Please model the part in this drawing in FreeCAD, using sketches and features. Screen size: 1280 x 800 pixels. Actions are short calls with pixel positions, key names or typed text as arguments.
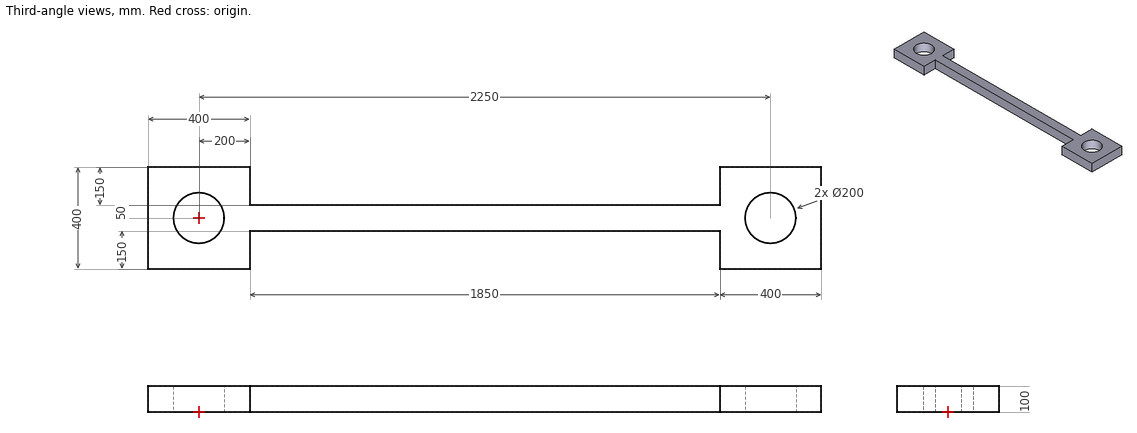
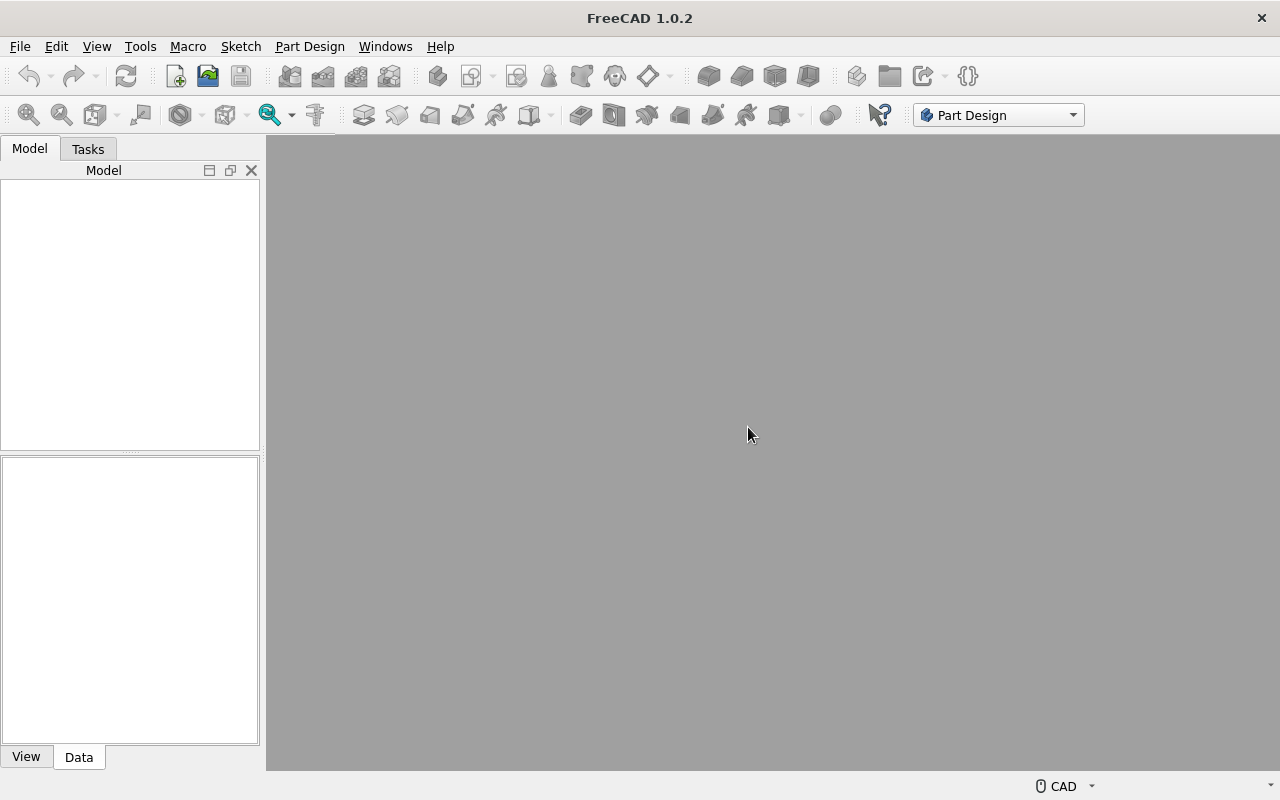
click(175, 76)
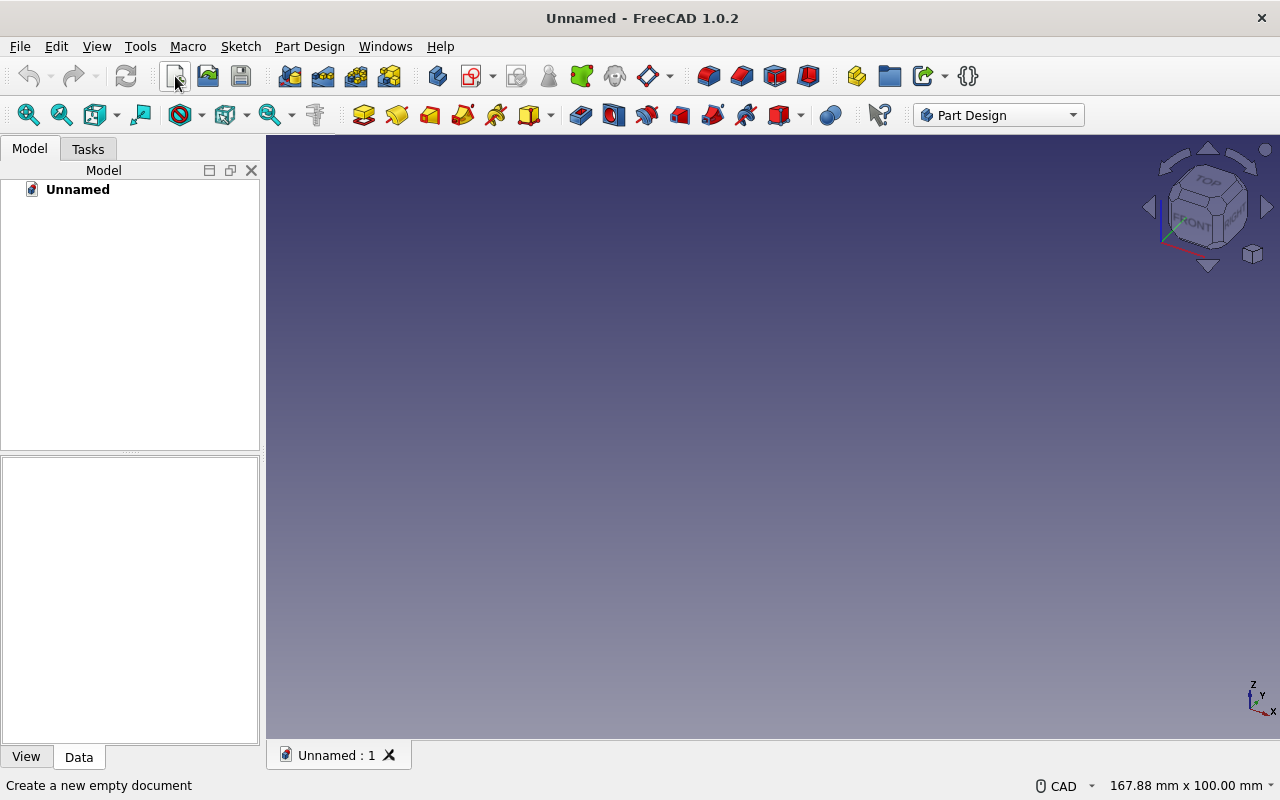
click(470, 76)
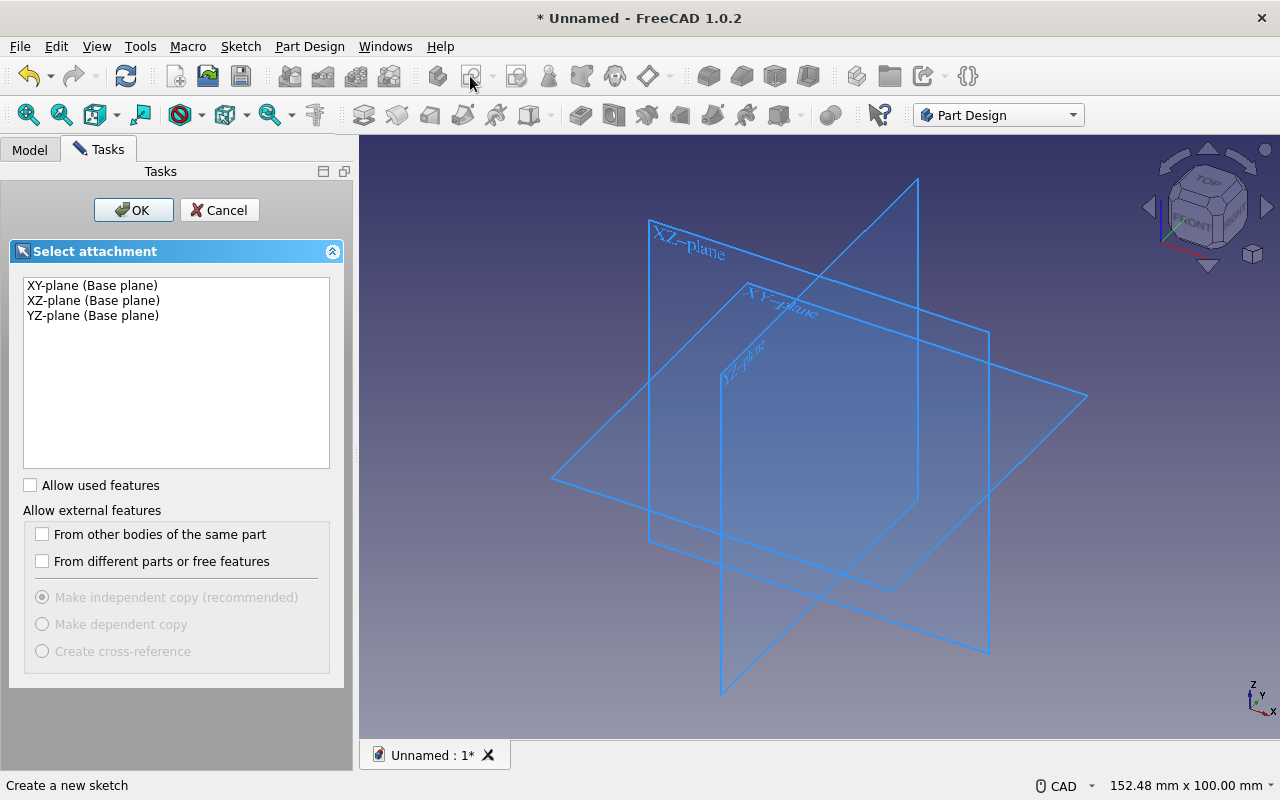
click(84, 286)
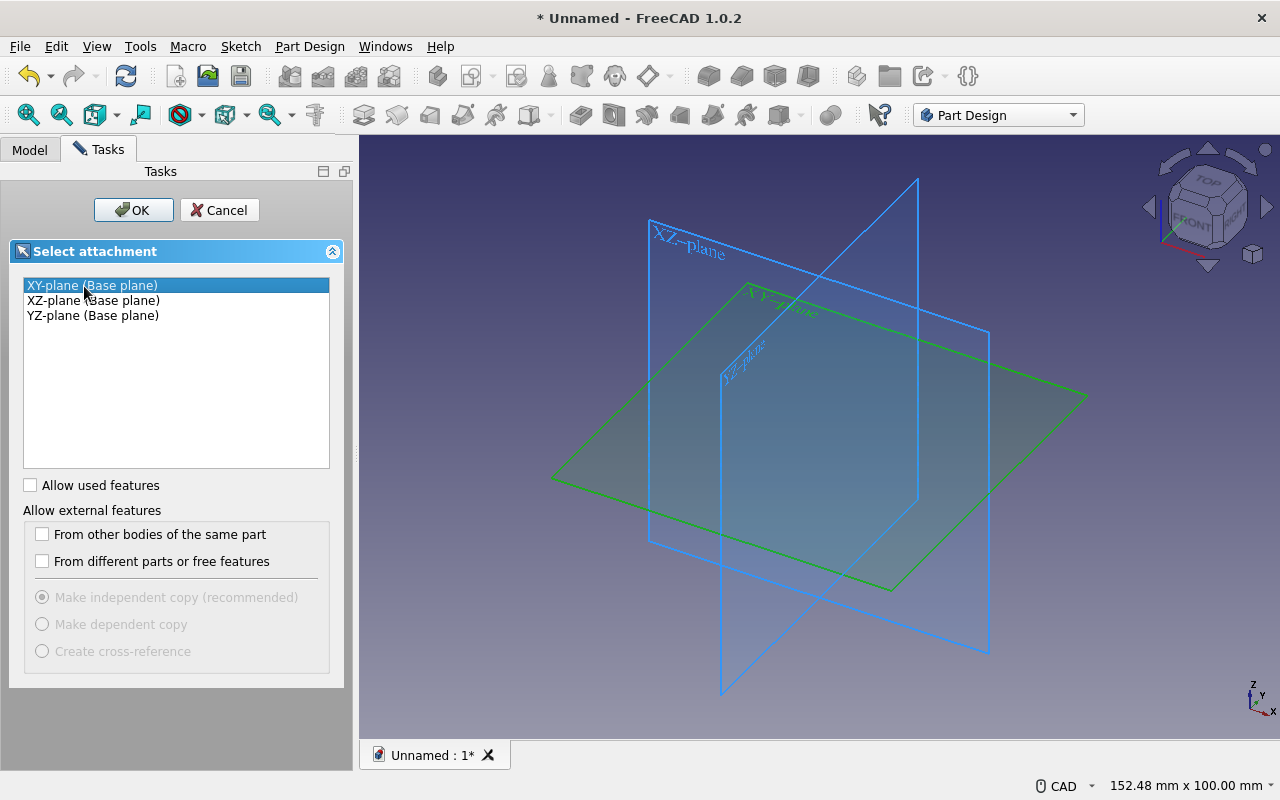
click(134, 210)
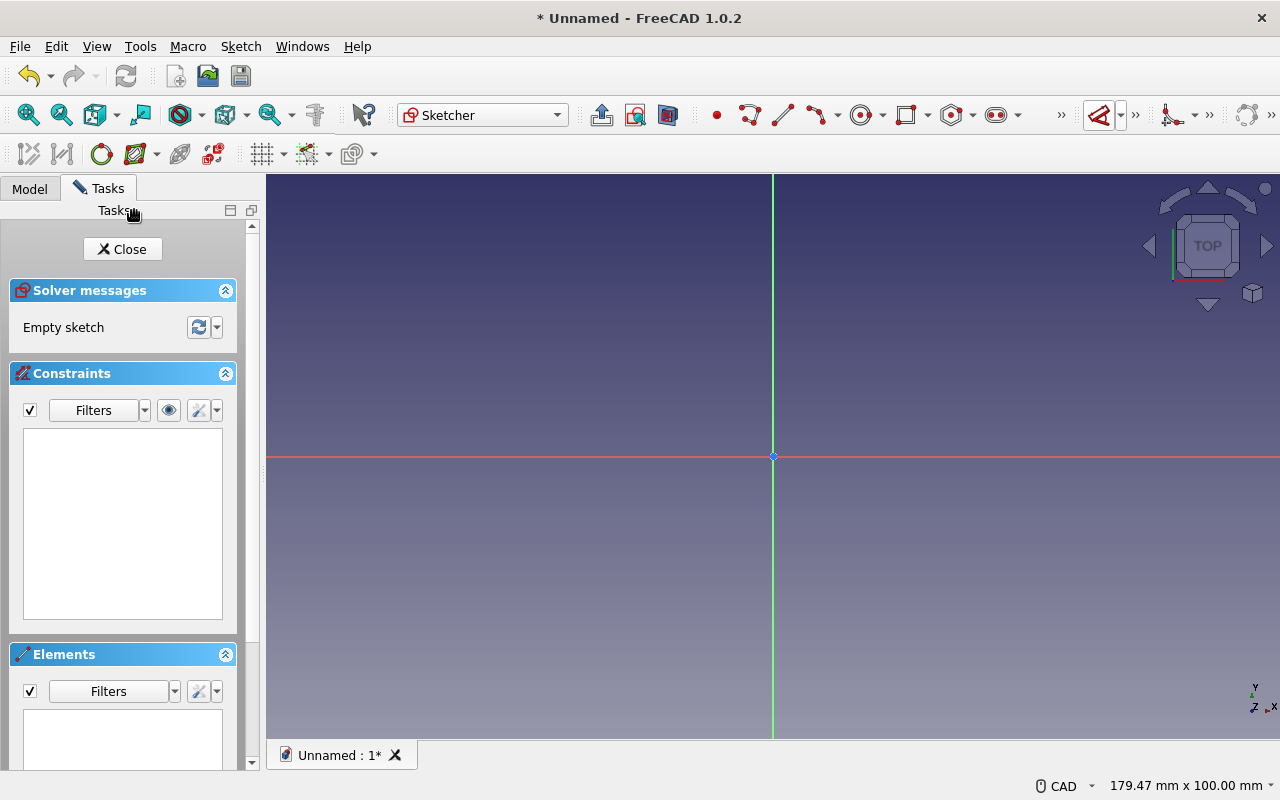
scroll(368, 457, down, 15)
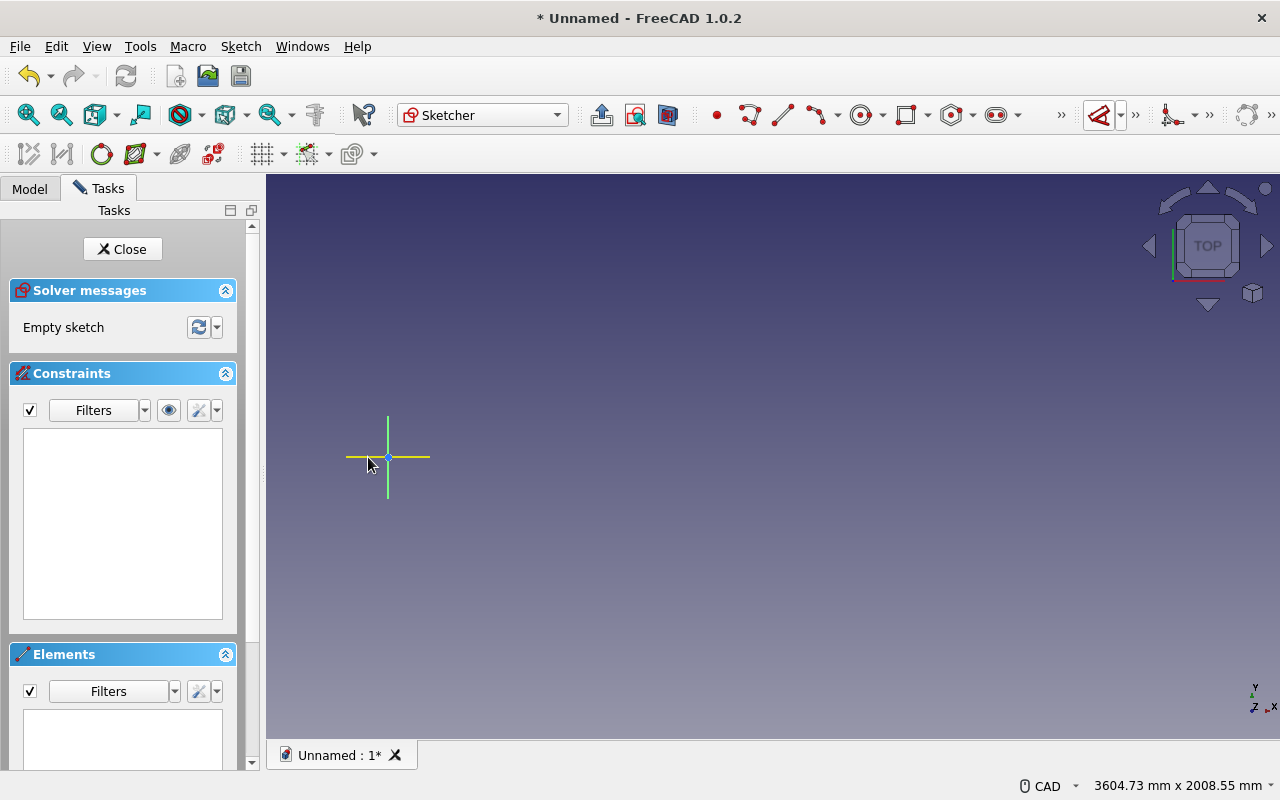
click(750, 116)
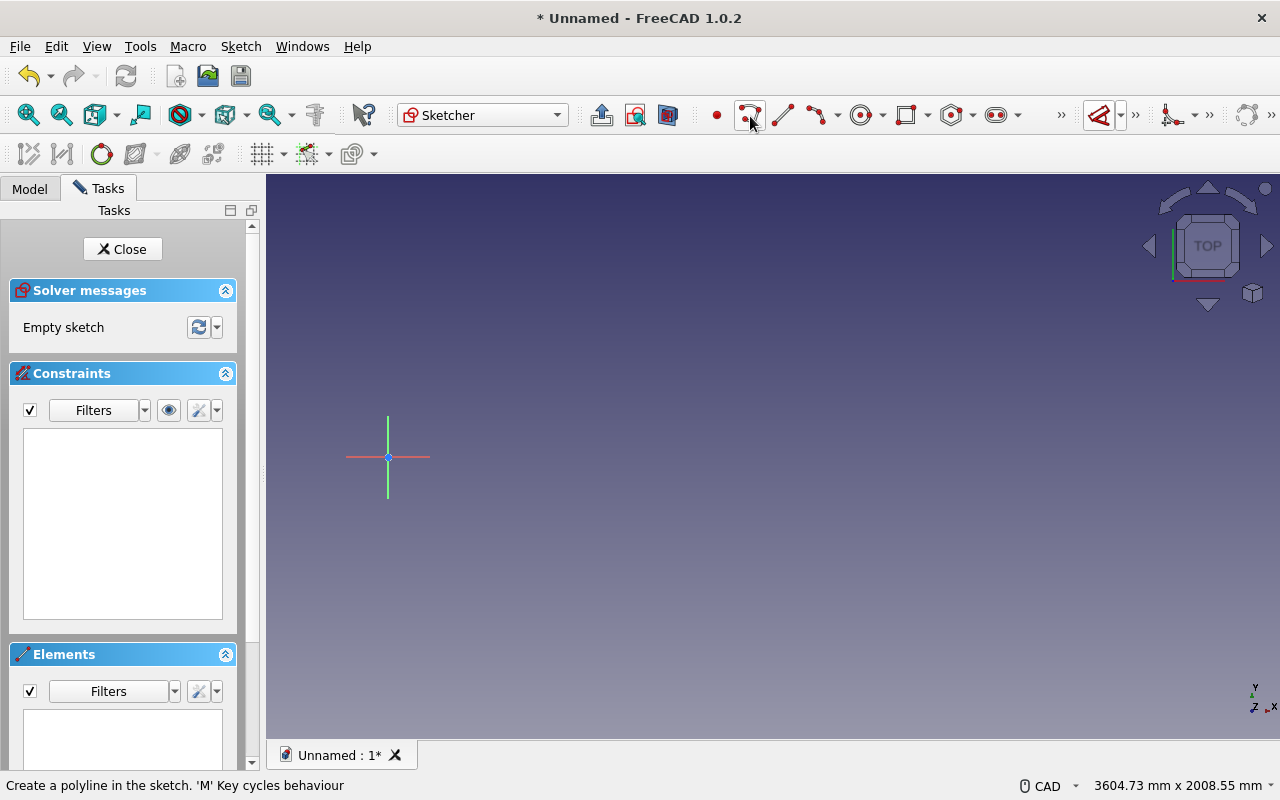
click(445, 443)
click(445, 401)
click(332, 401)
click(332, 514)
click(445, 514)
click(445, 472)
click(965, 472)
click(965, 514)
click(1077, 514)
click(1077, 401)
click(965, 401)
click(965, 443)
click(445, 444)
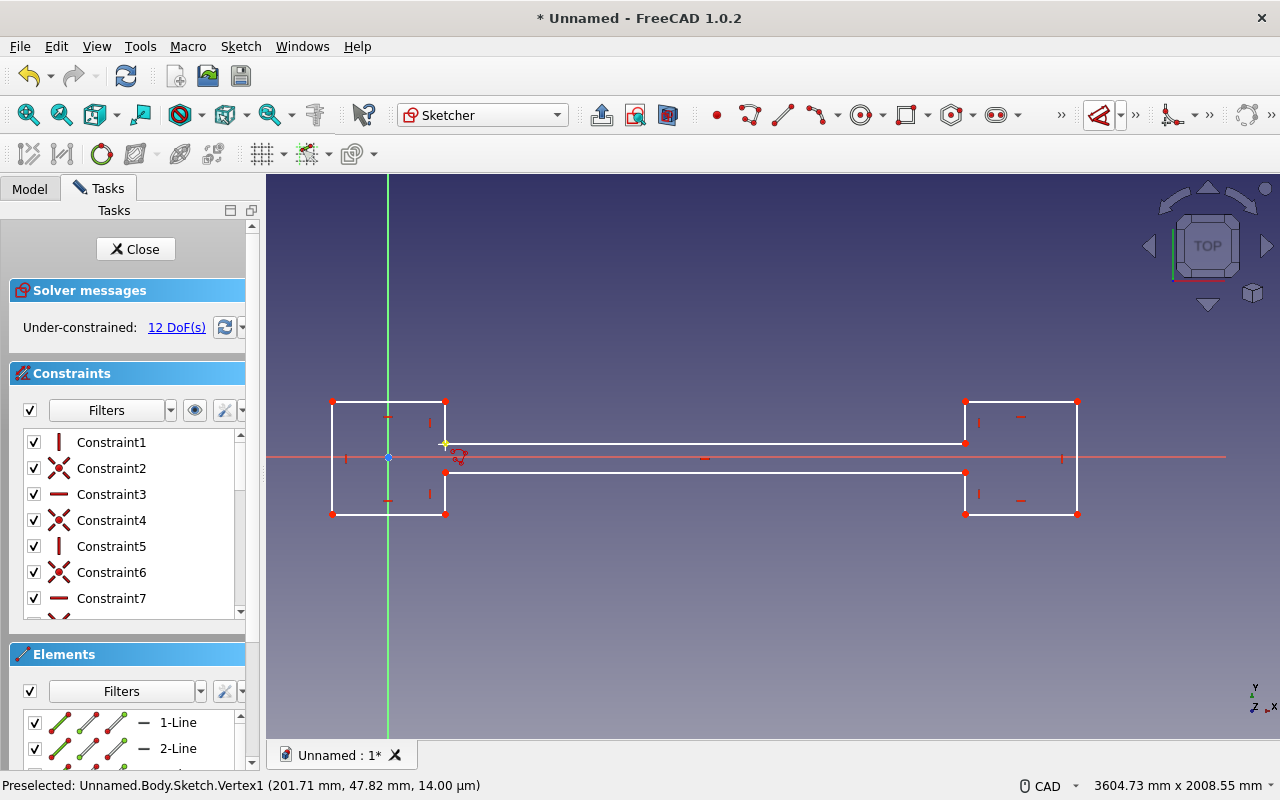
click(860, 116)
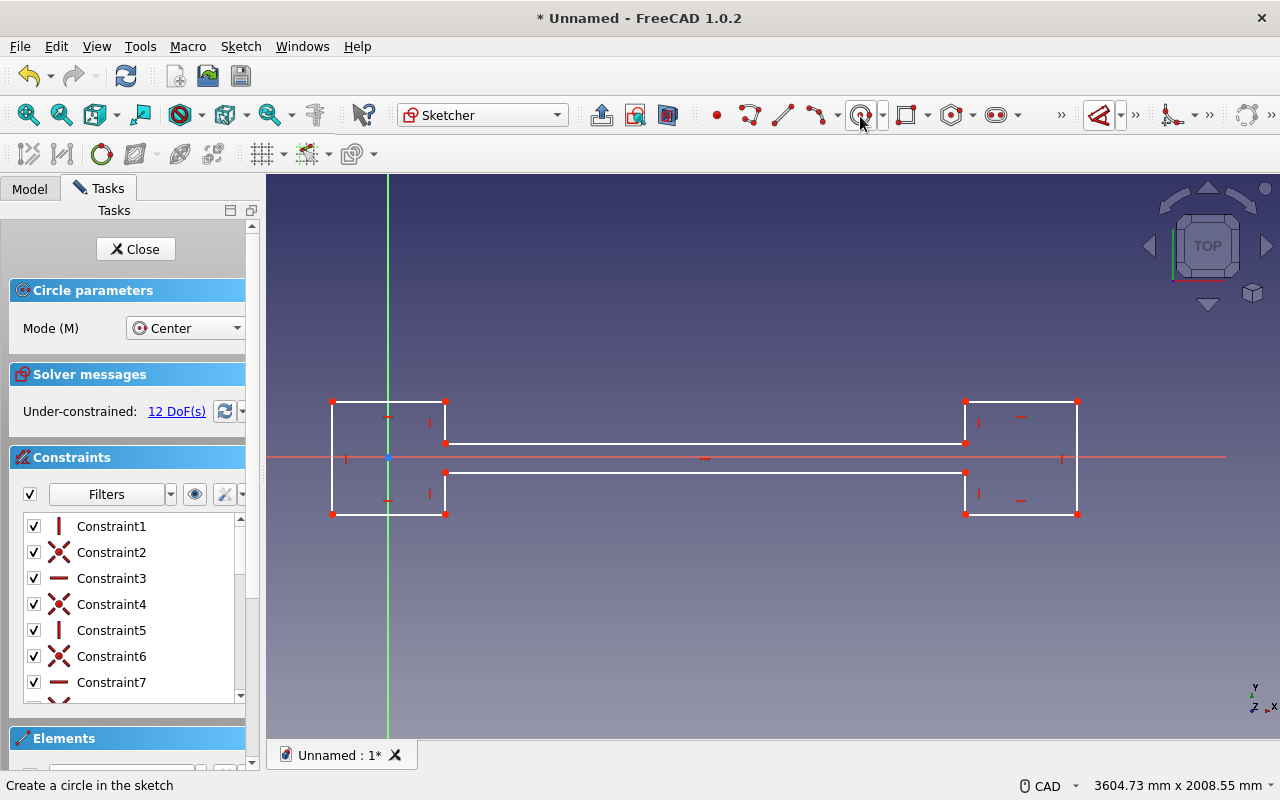
click(1021, 457)
click(1041, 438)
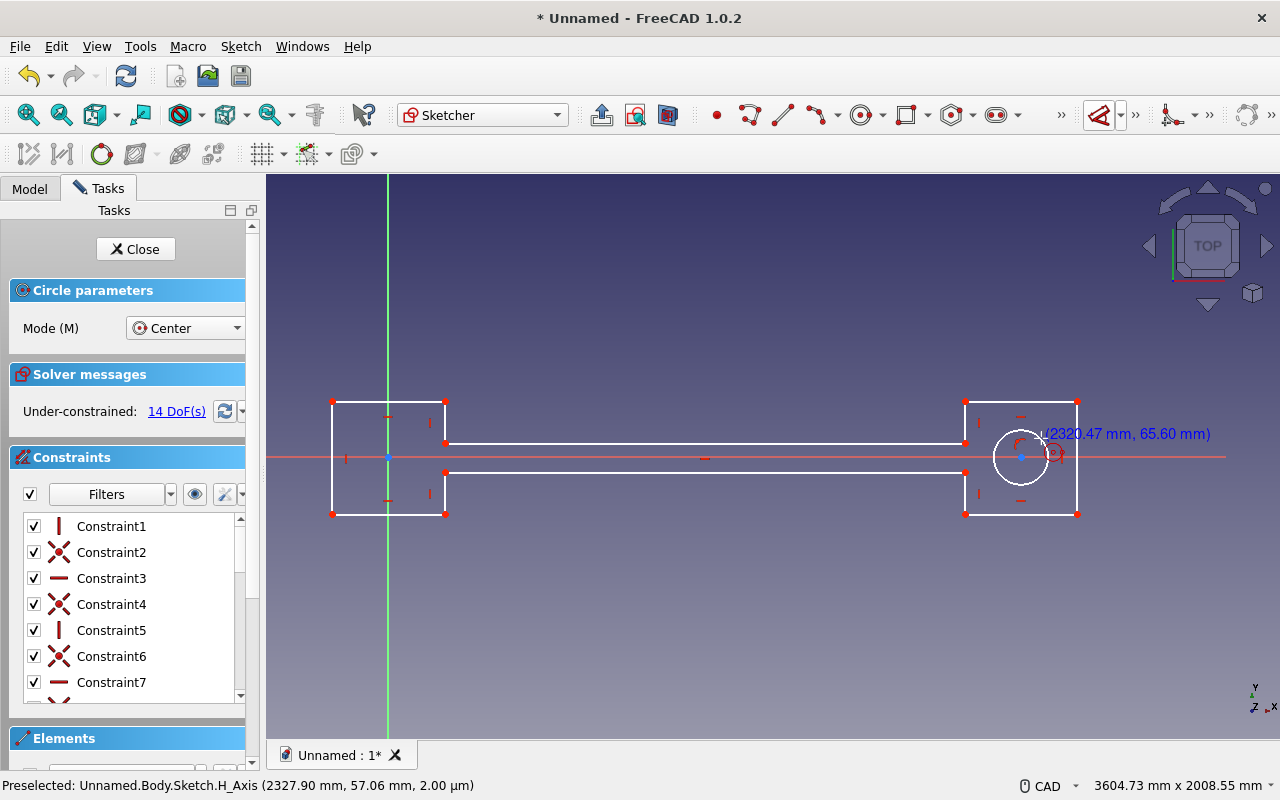
click(388, 457)
click(408, 438)
key(Escape)